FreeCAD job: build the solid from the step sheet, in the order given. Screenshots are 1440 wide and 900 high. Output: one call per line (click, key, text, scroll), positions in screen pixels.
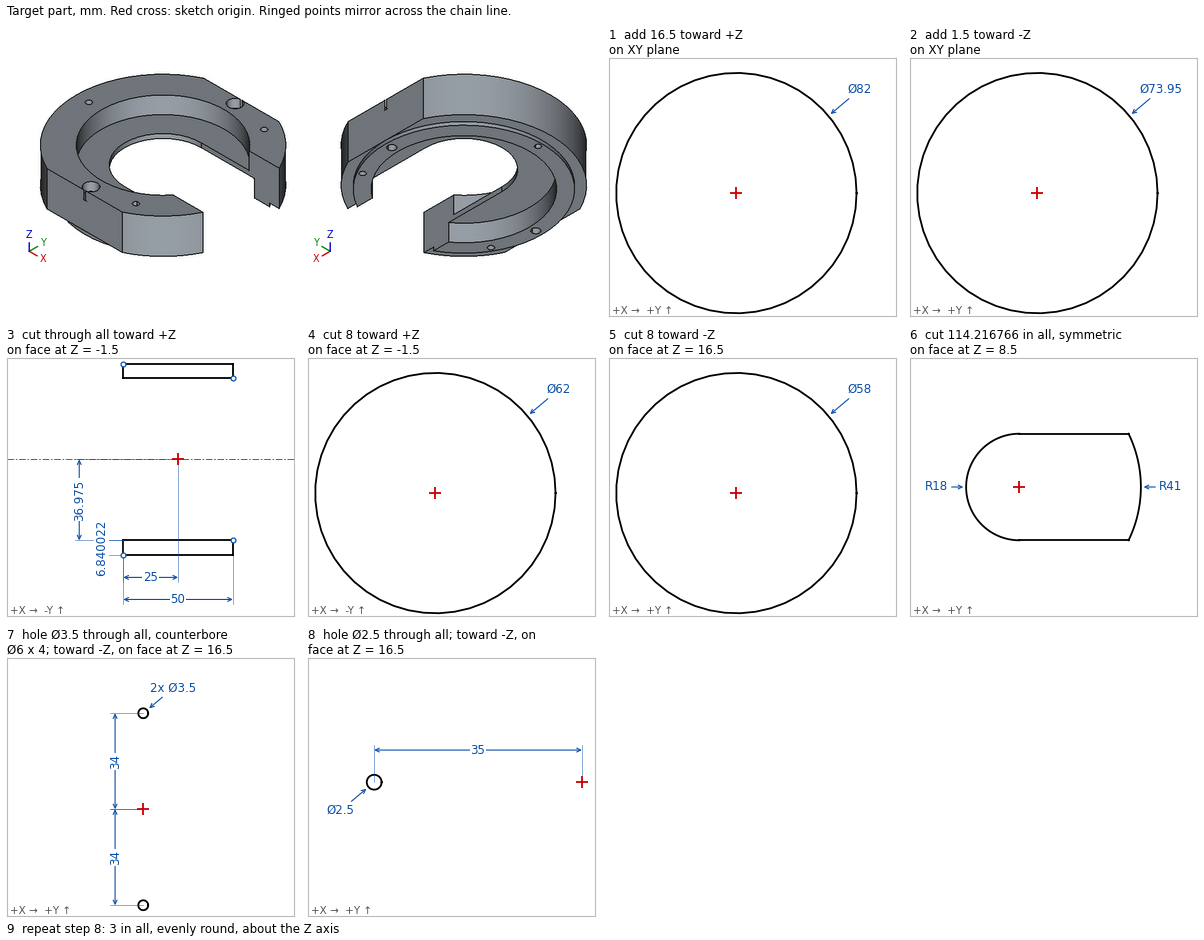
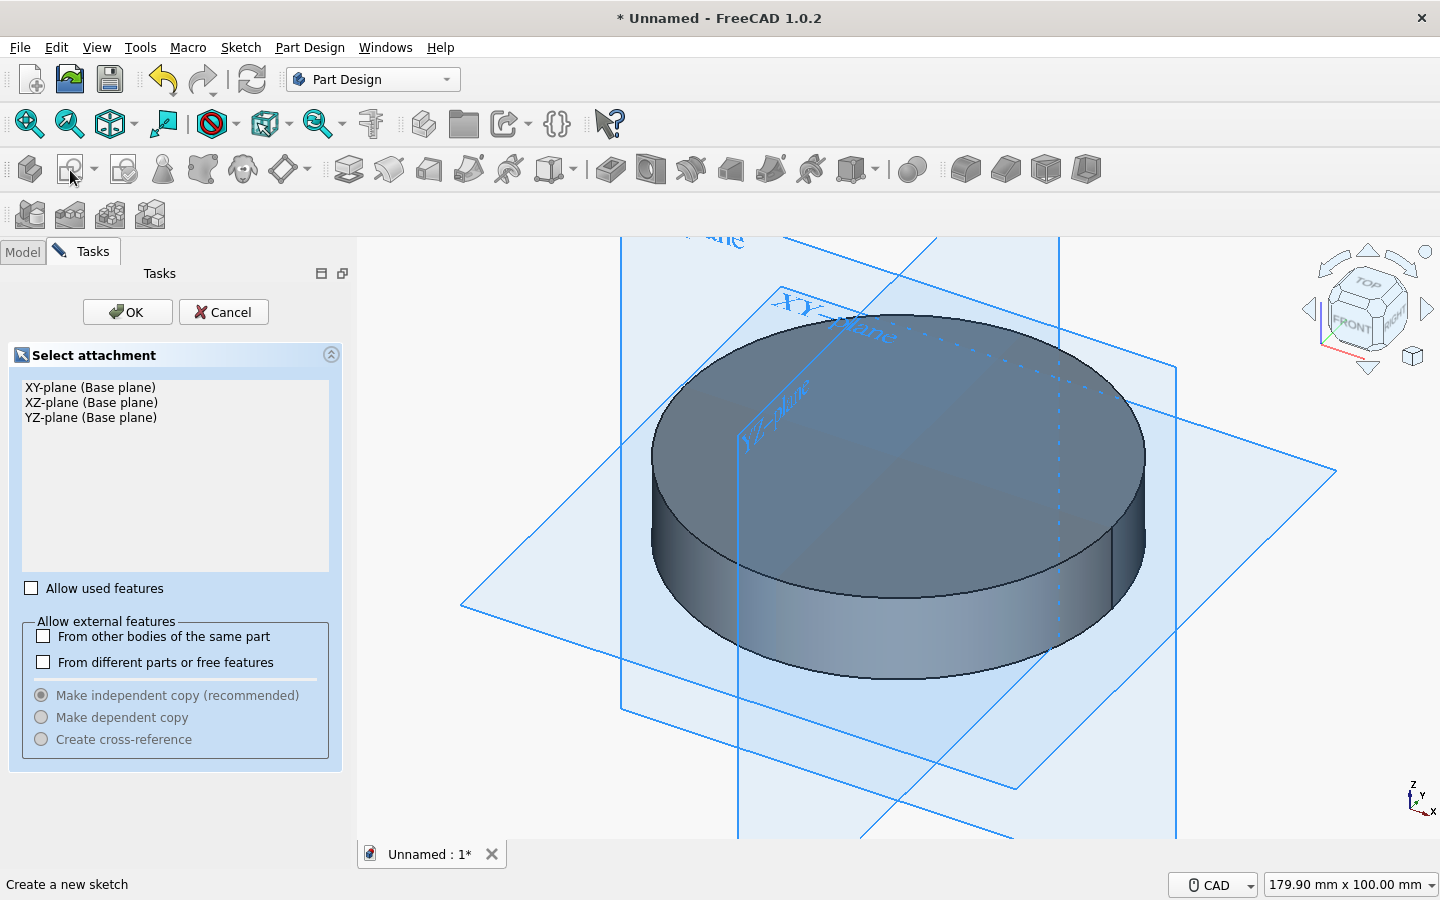
click(82, 388)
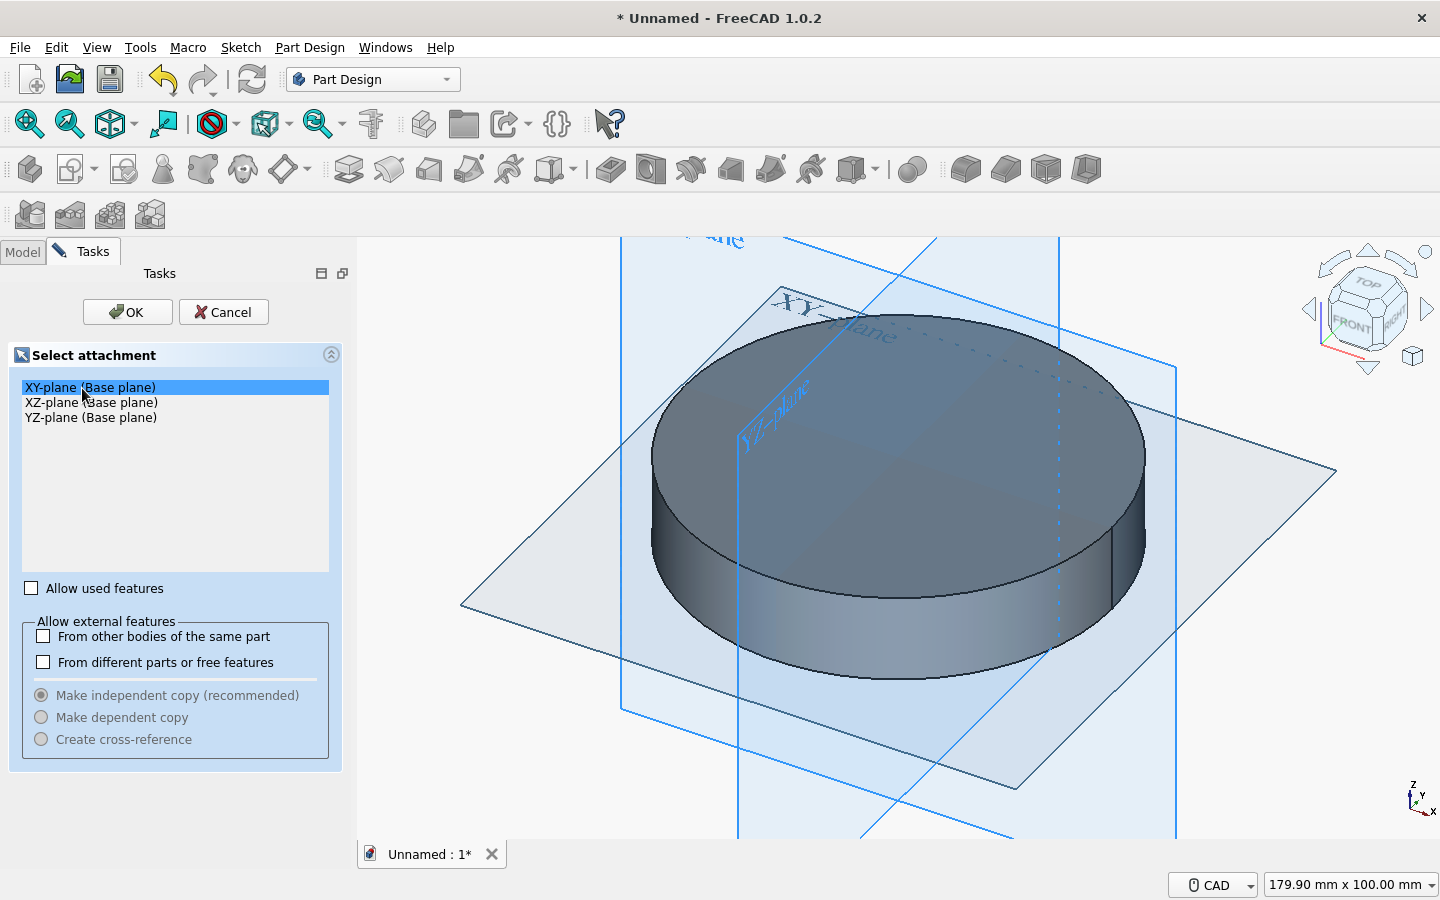
click(128, 312)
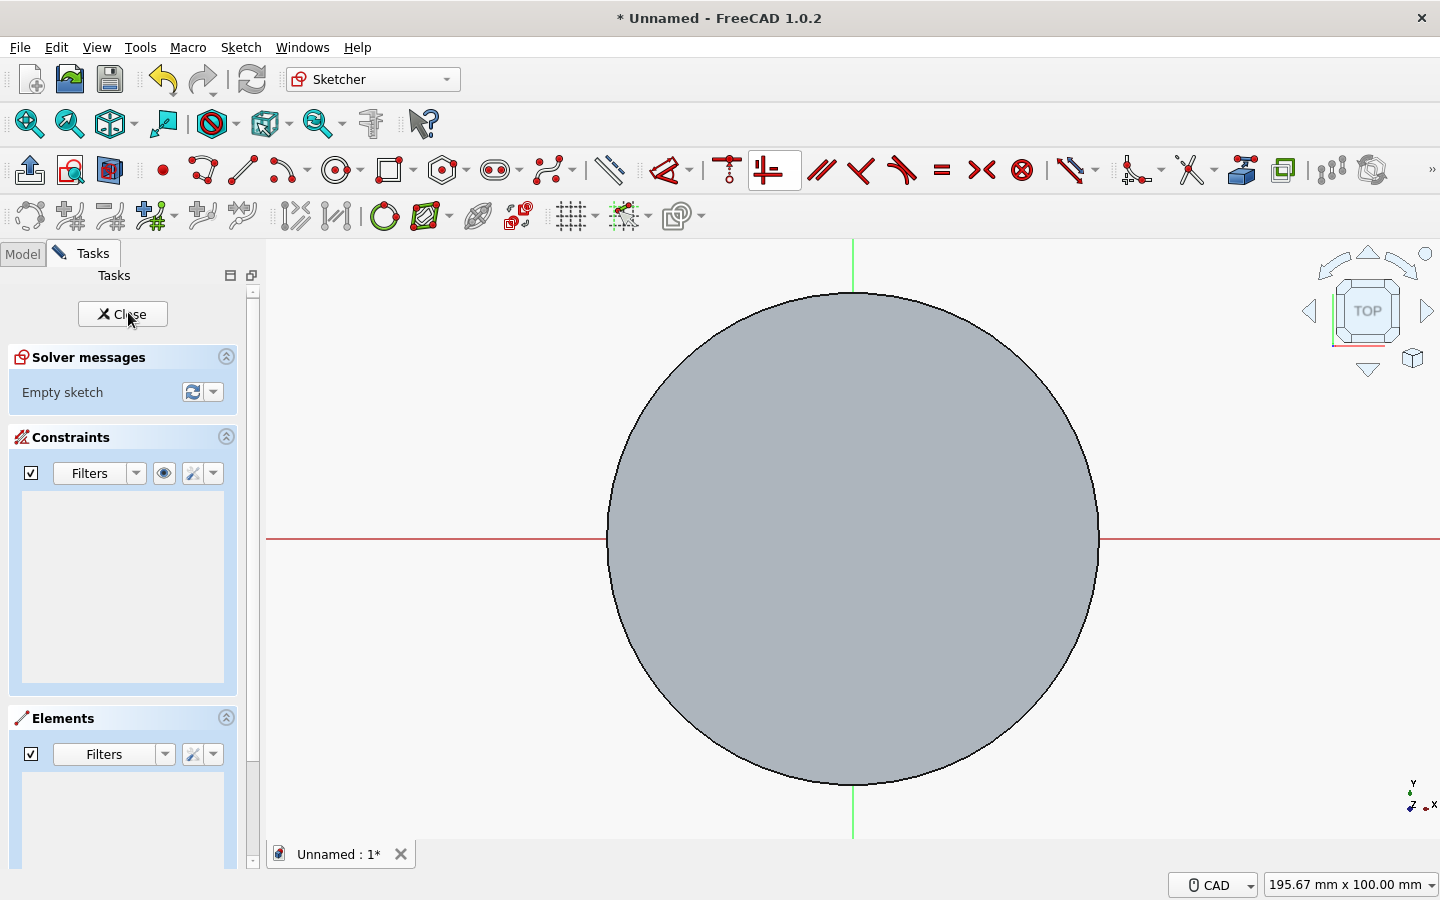
key(q)
key(s)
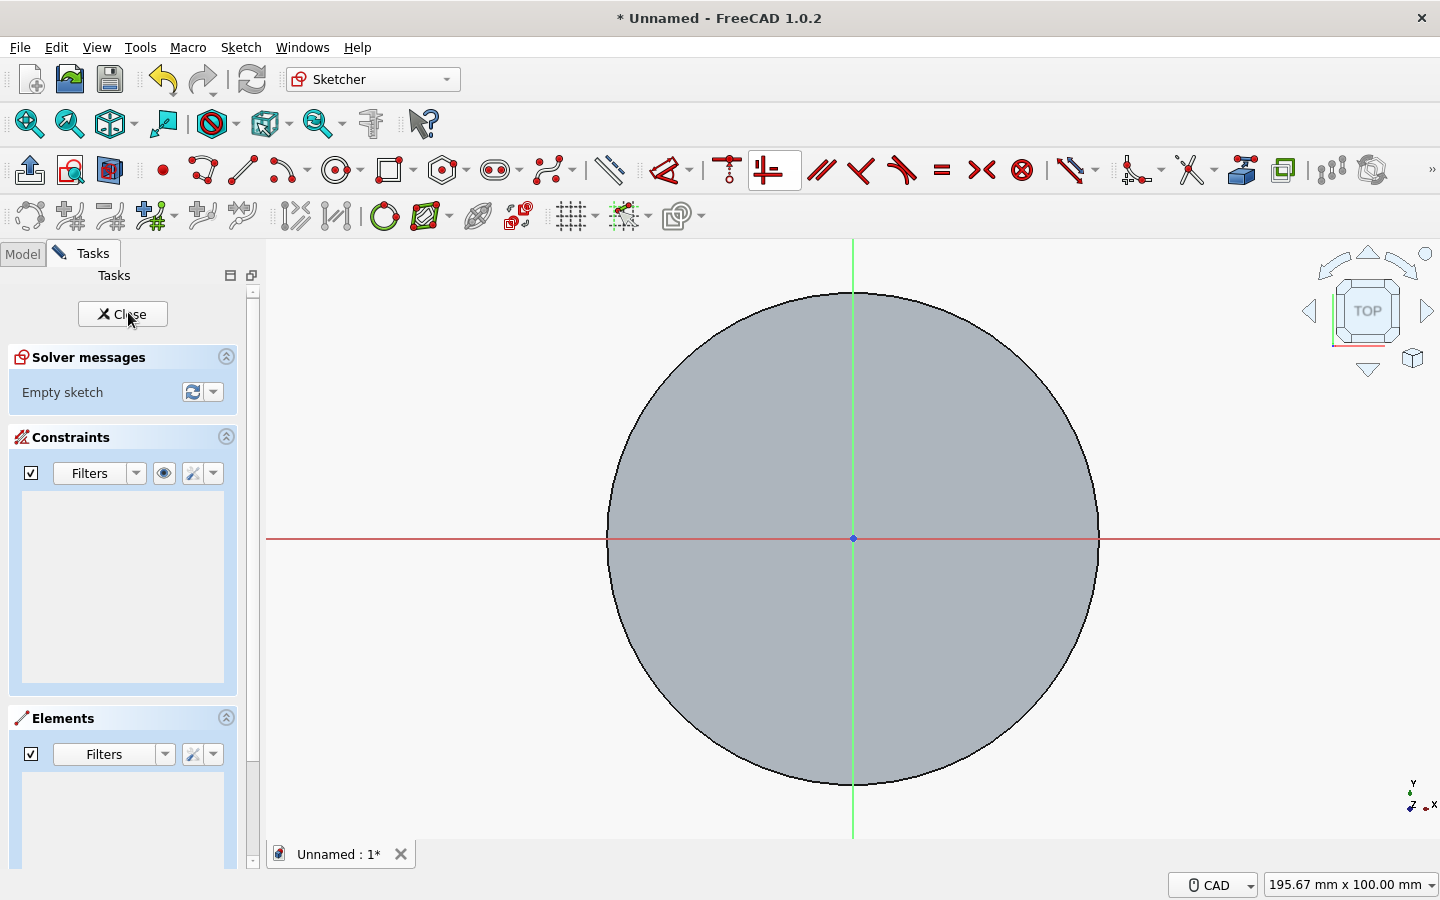
key(g)
key(c)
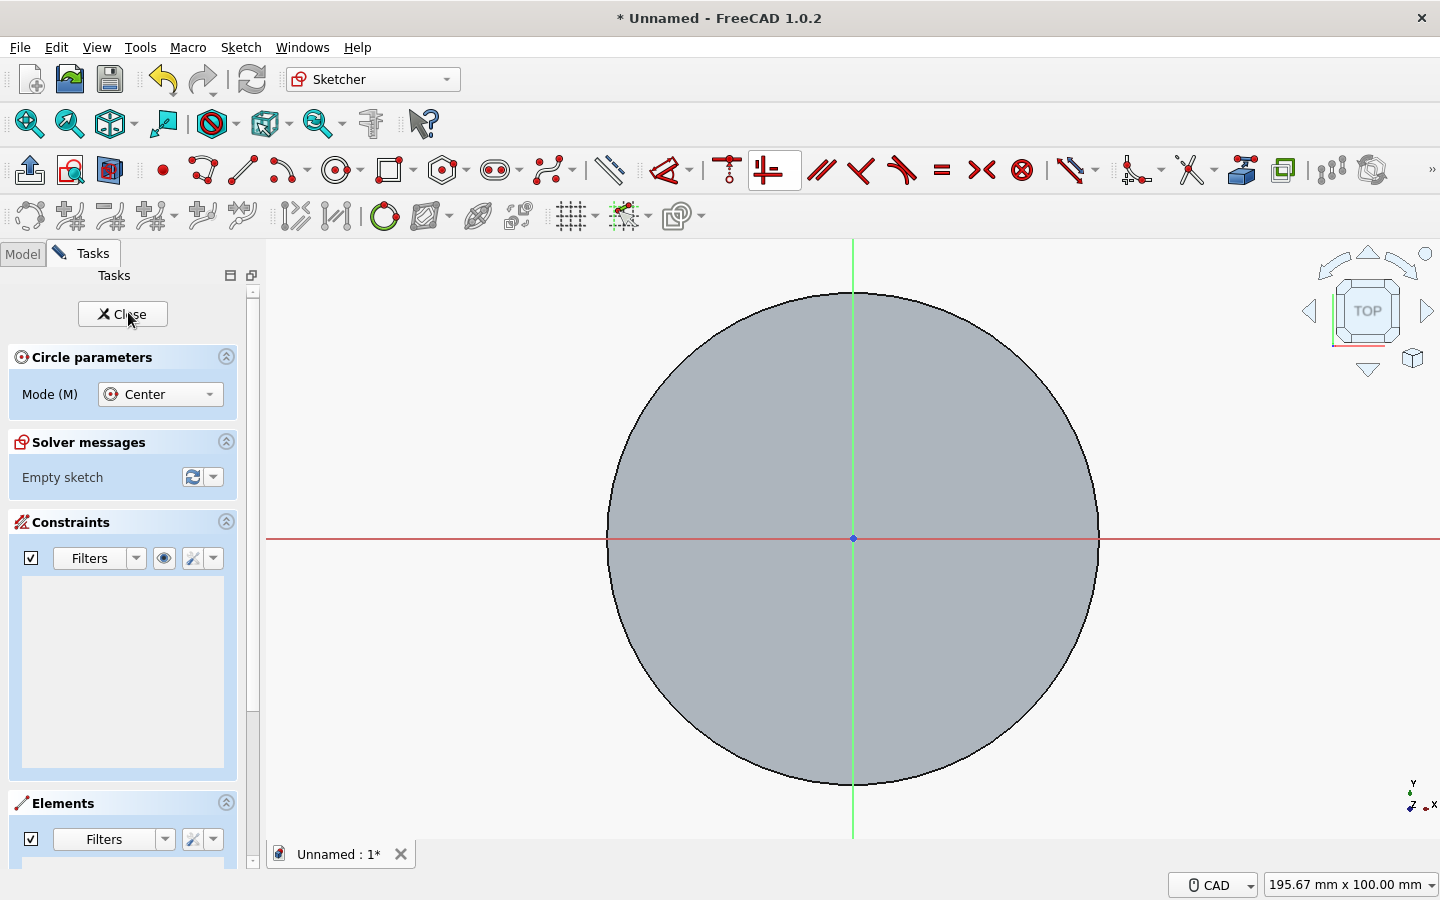
click(853, 539)
click(1010, 382)
key(Escape)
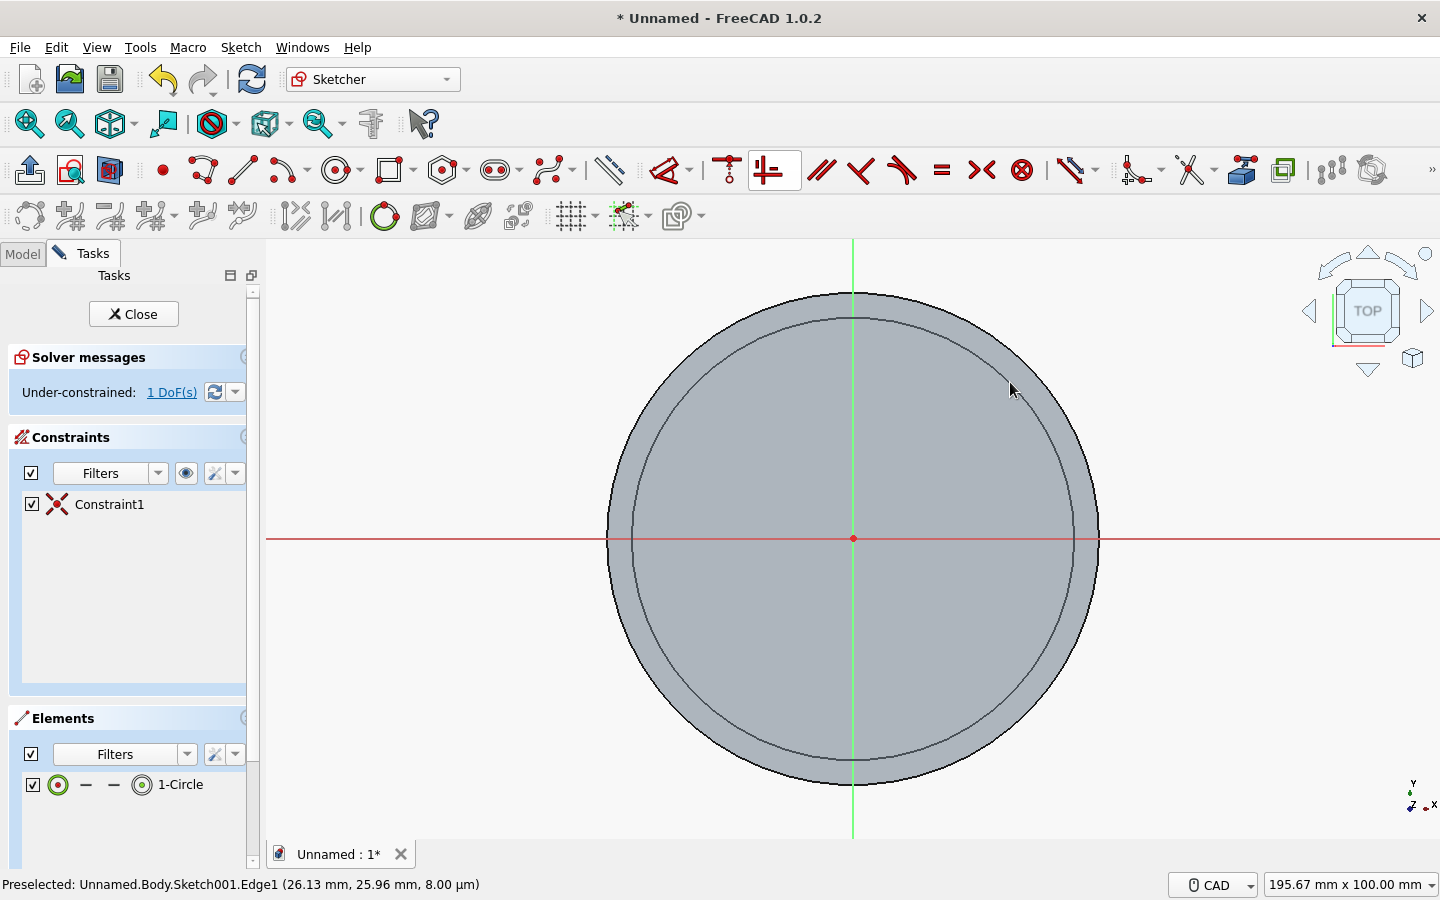
key(d)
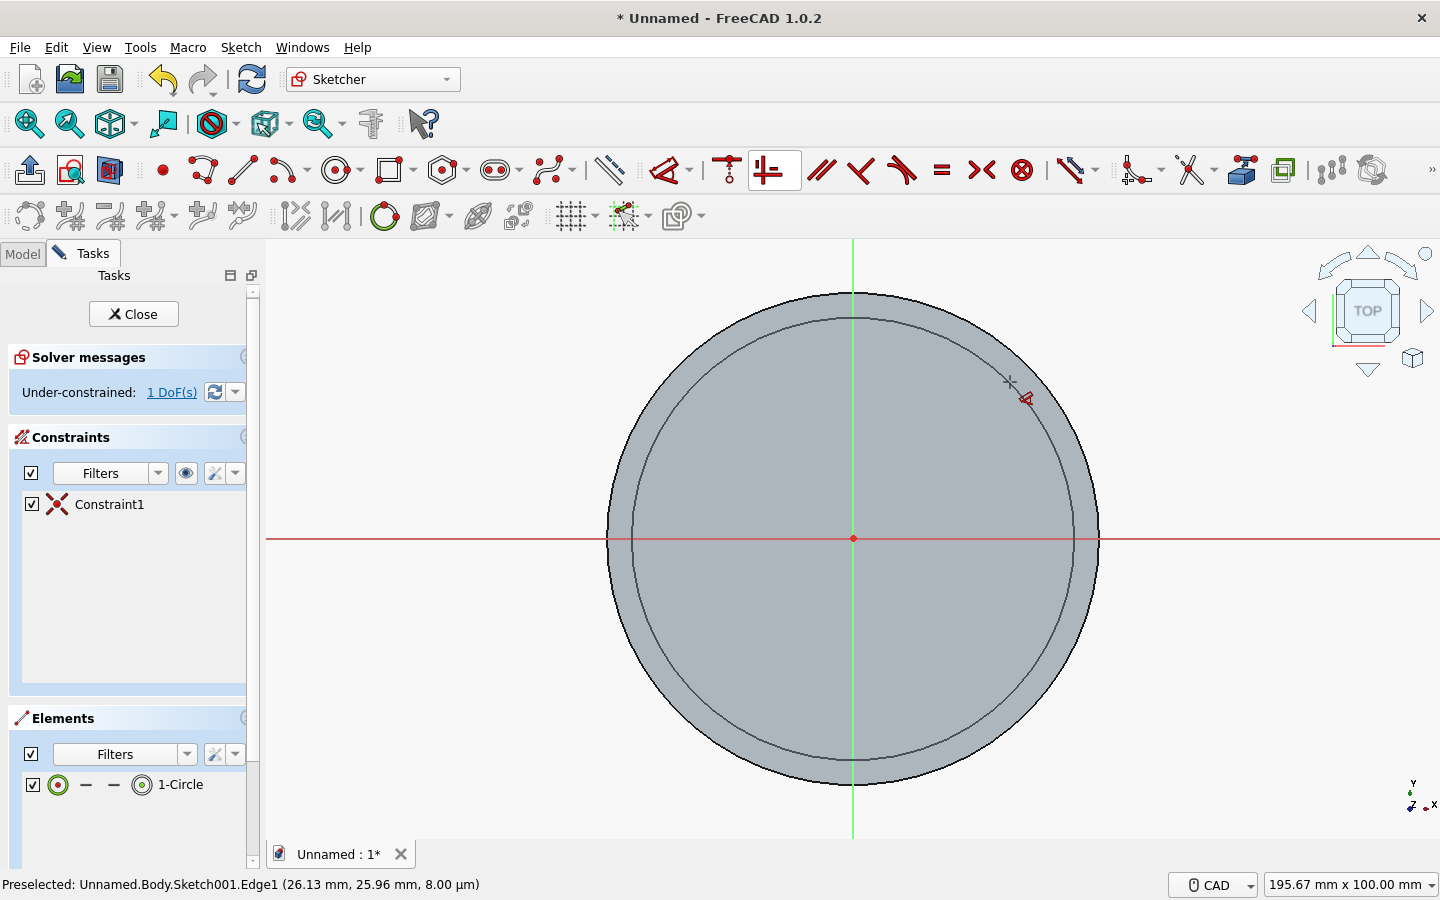
click(1009, 382)
click(1032, 359)